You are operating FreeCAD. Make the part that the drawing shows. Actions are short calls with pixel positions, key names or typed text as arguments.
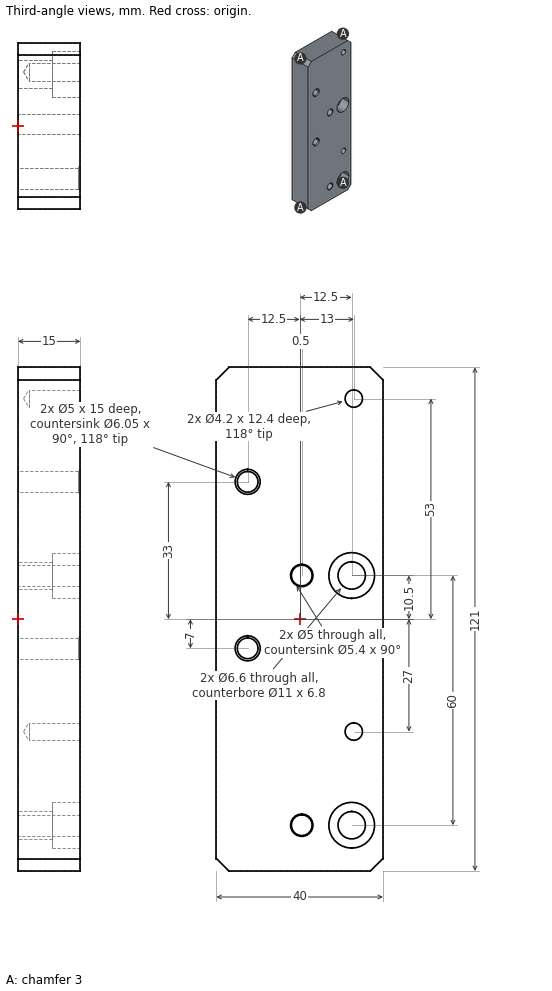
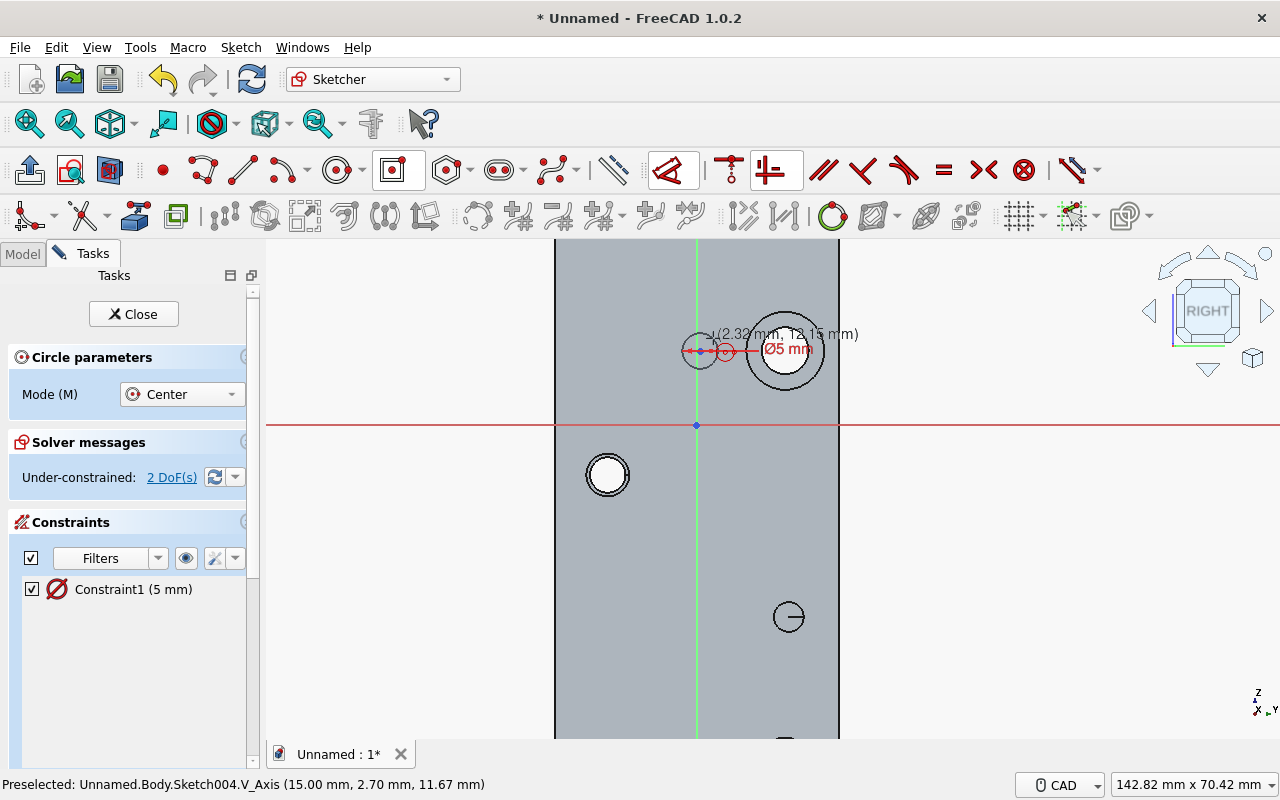
scroll(713, 337, down, 2)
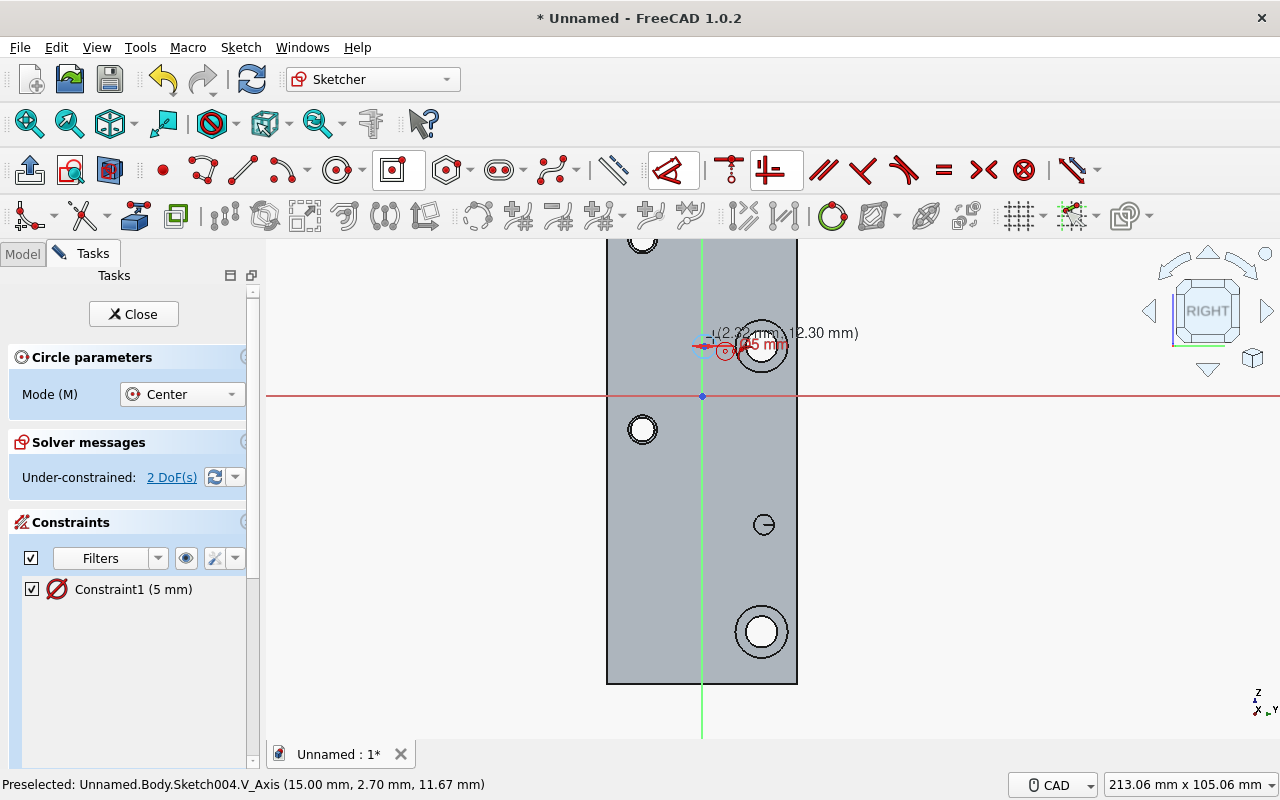
scroll(704, 632, up, 10)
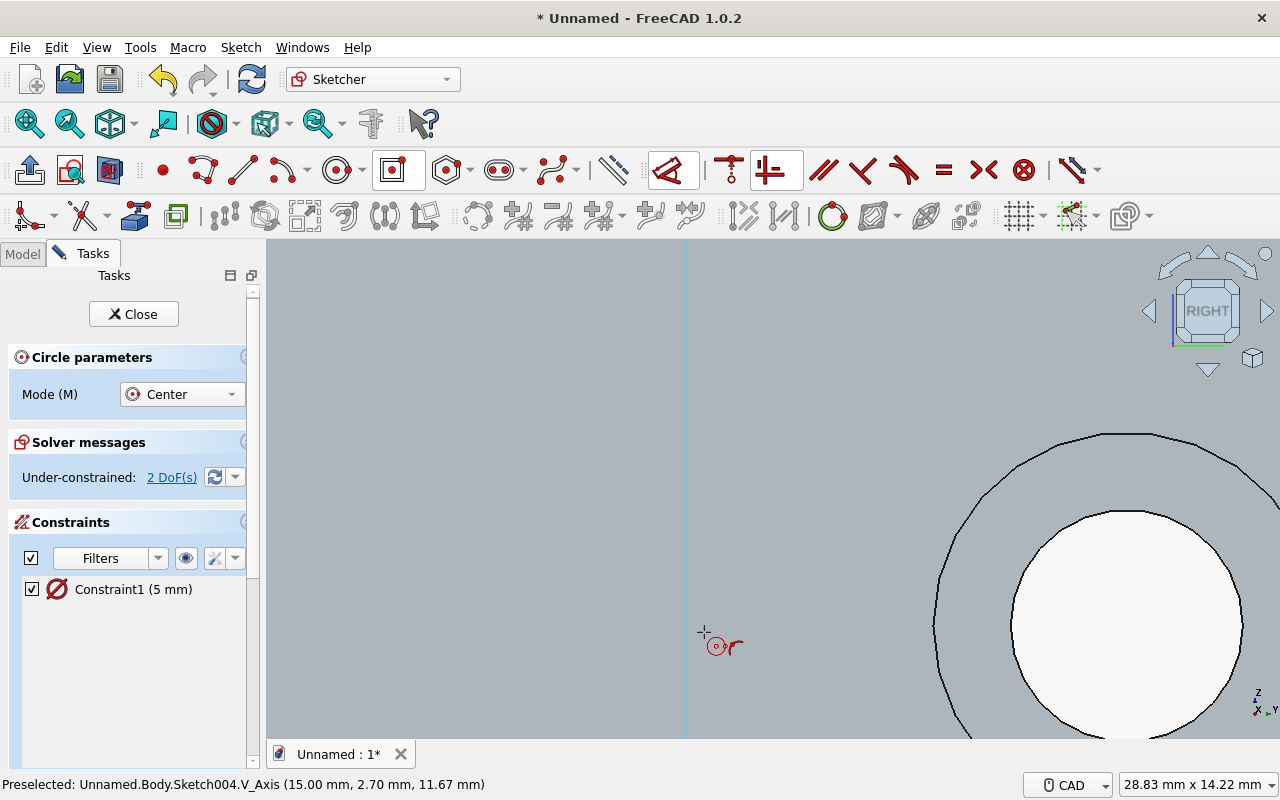
click(705, 626)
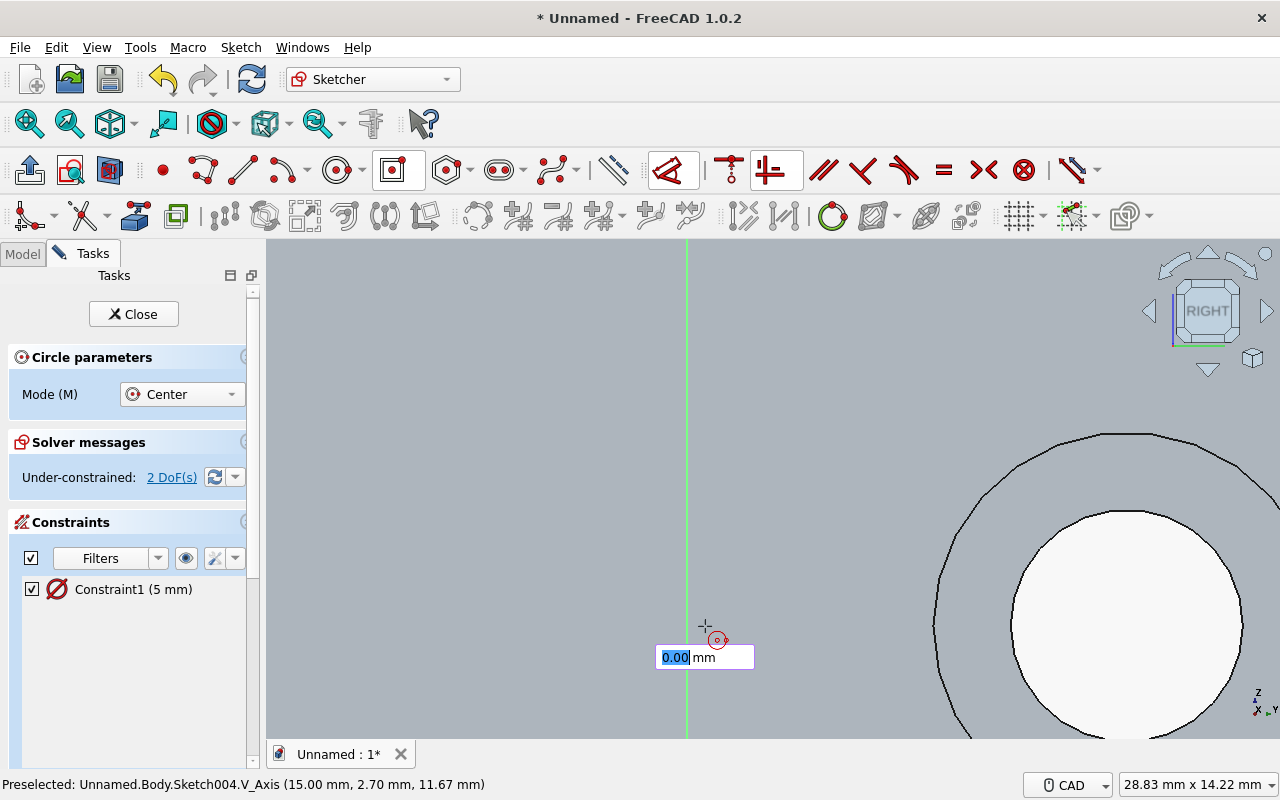
scroll(704, 633, down, 10)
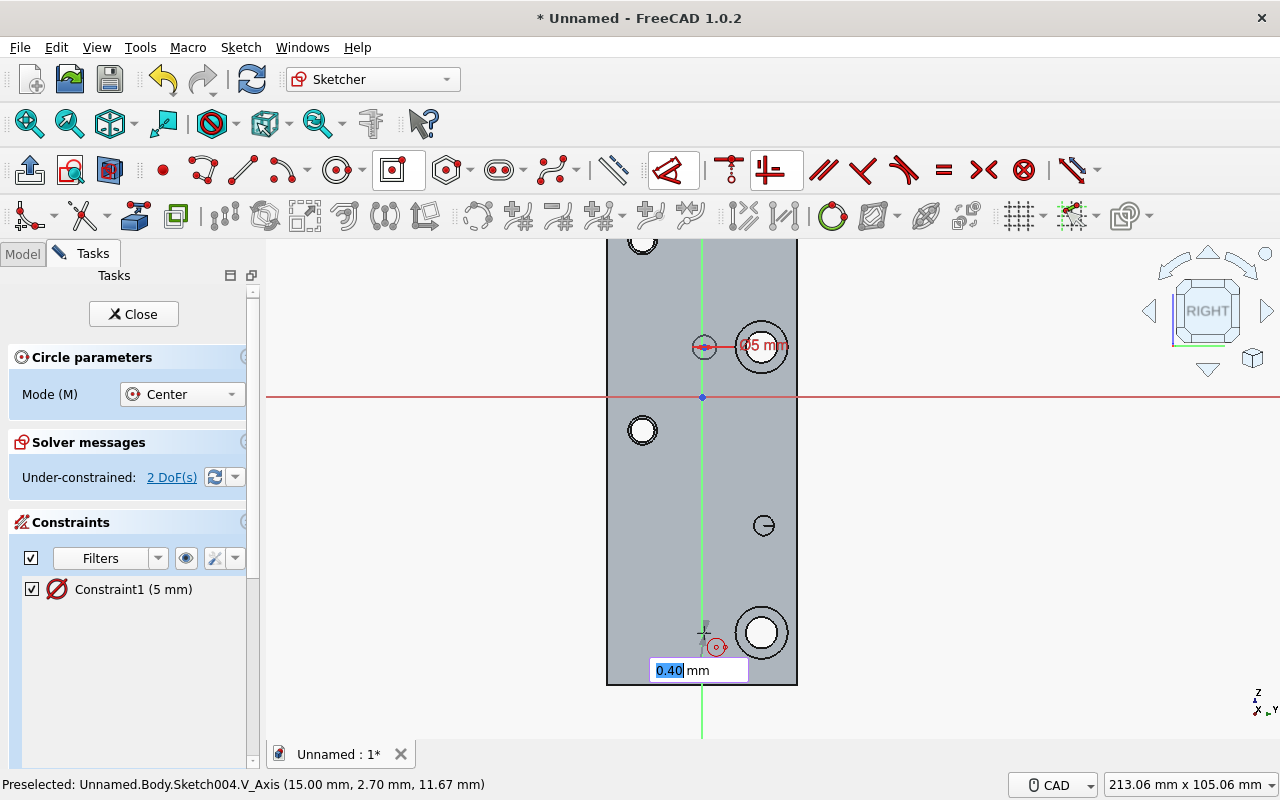
scroll(713, 624, up, 2)
move(713, 624)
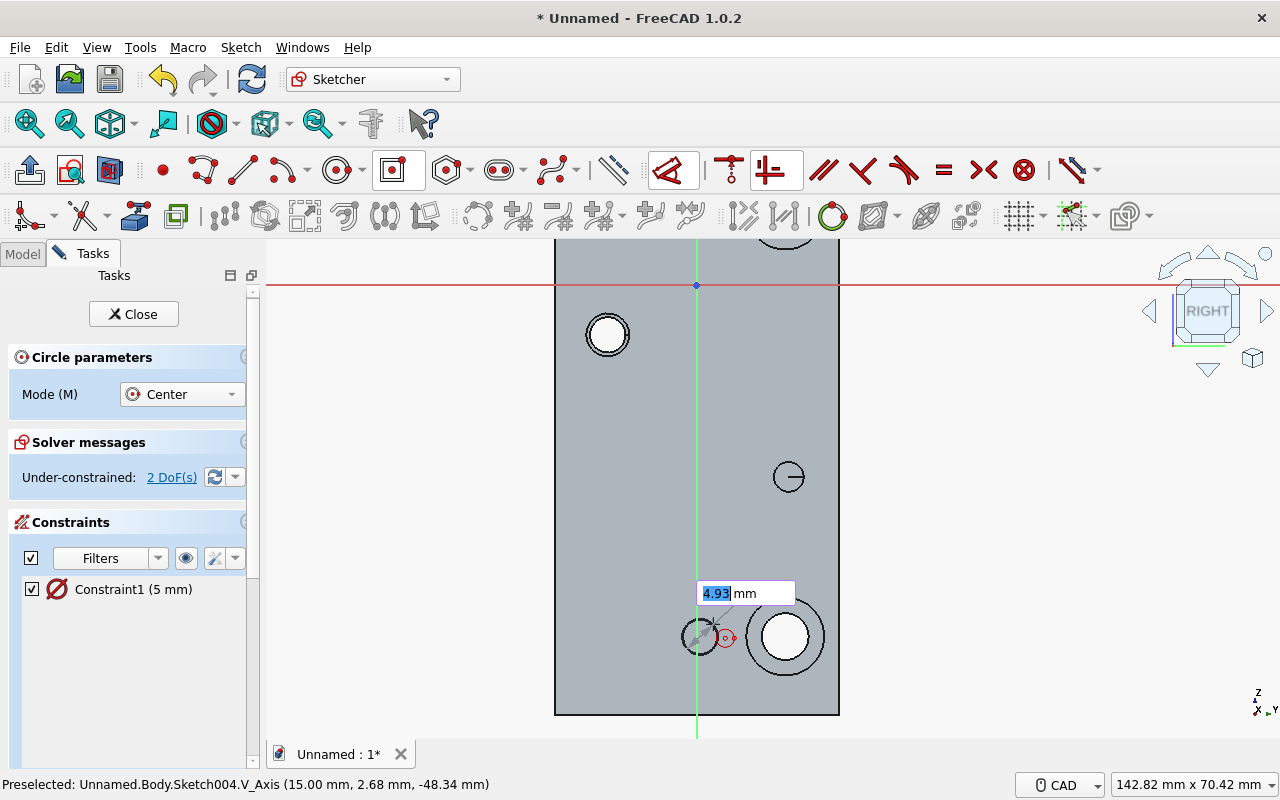
text(5)
key(Return)
key(Escape)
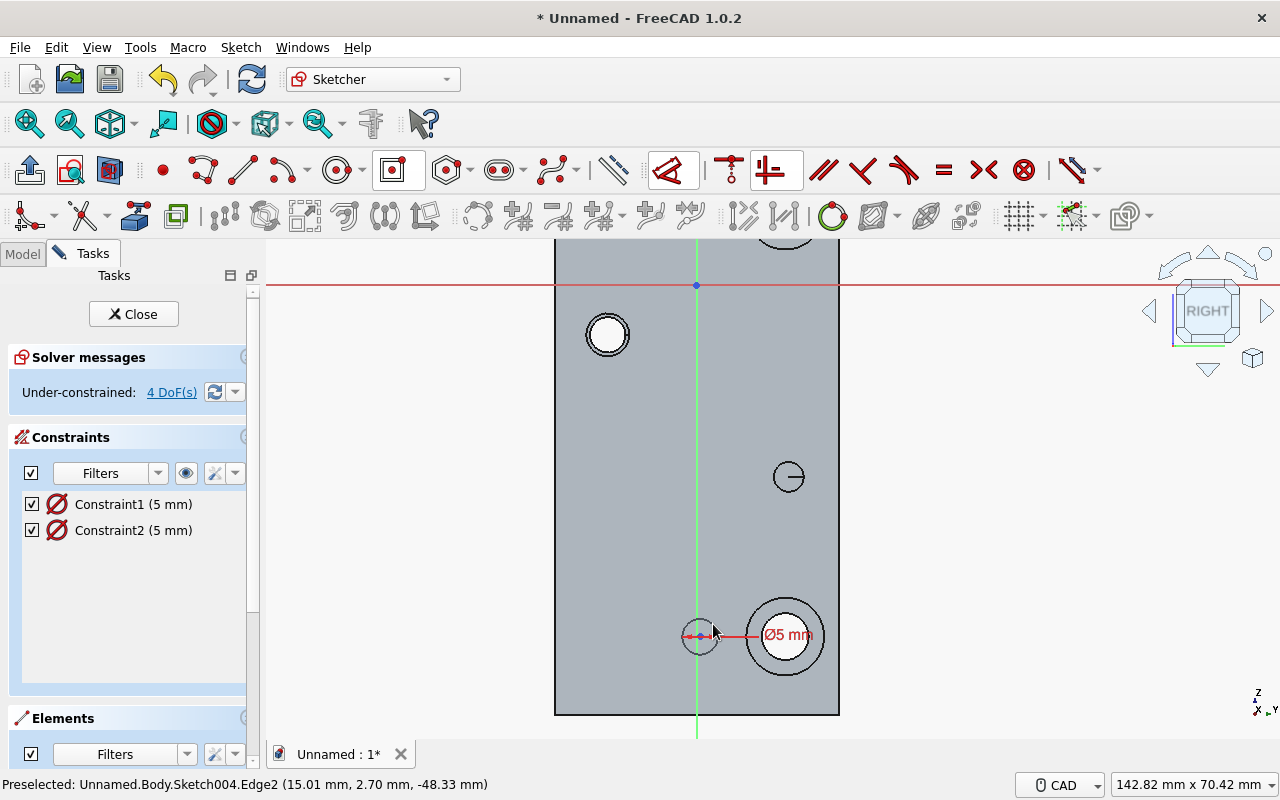
scroll(713, 622, down, 2)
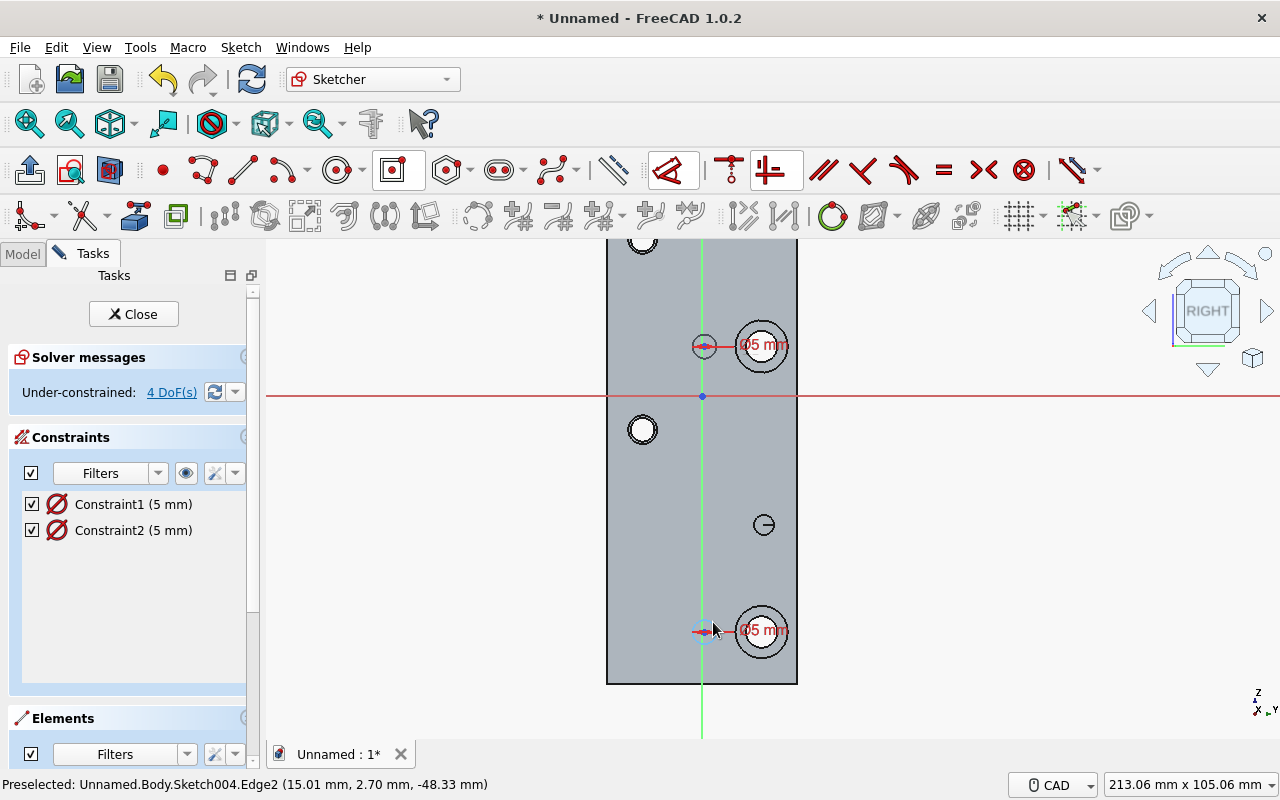
click(705, 347)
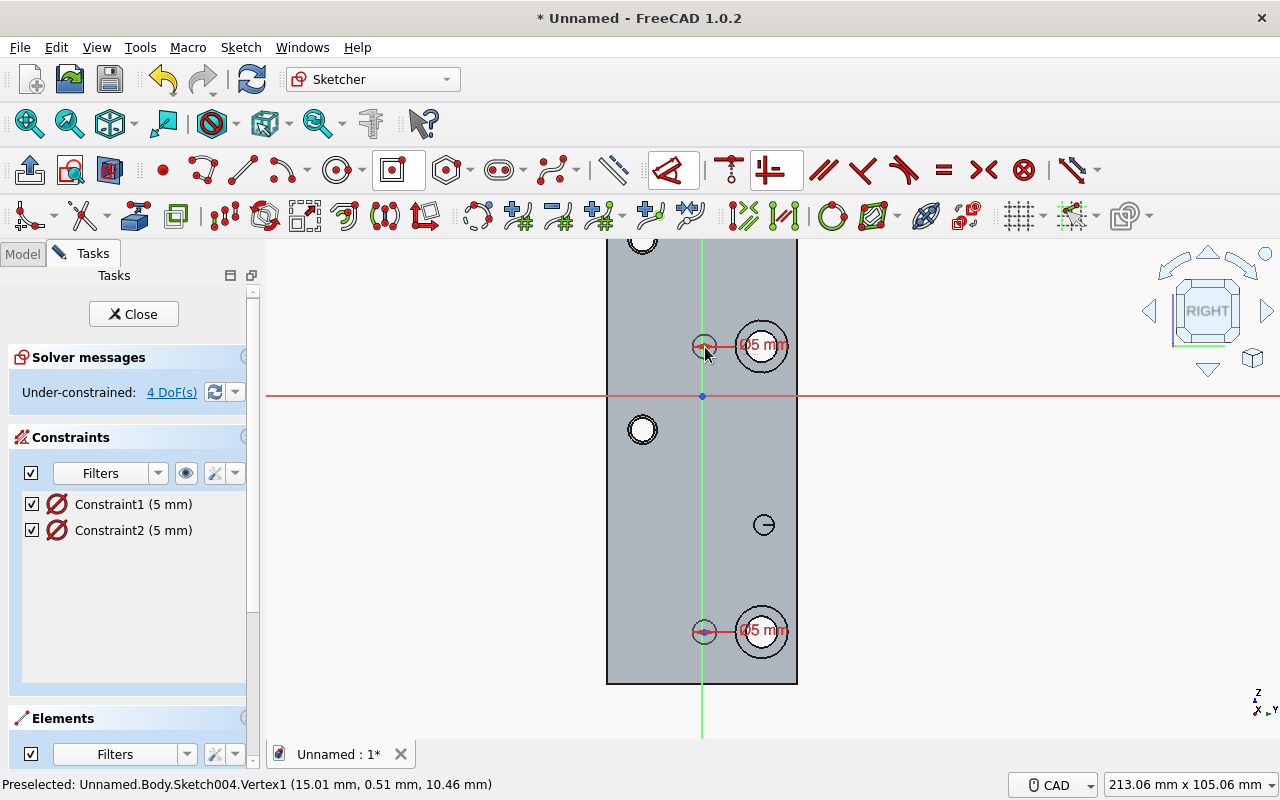
click(705, 632)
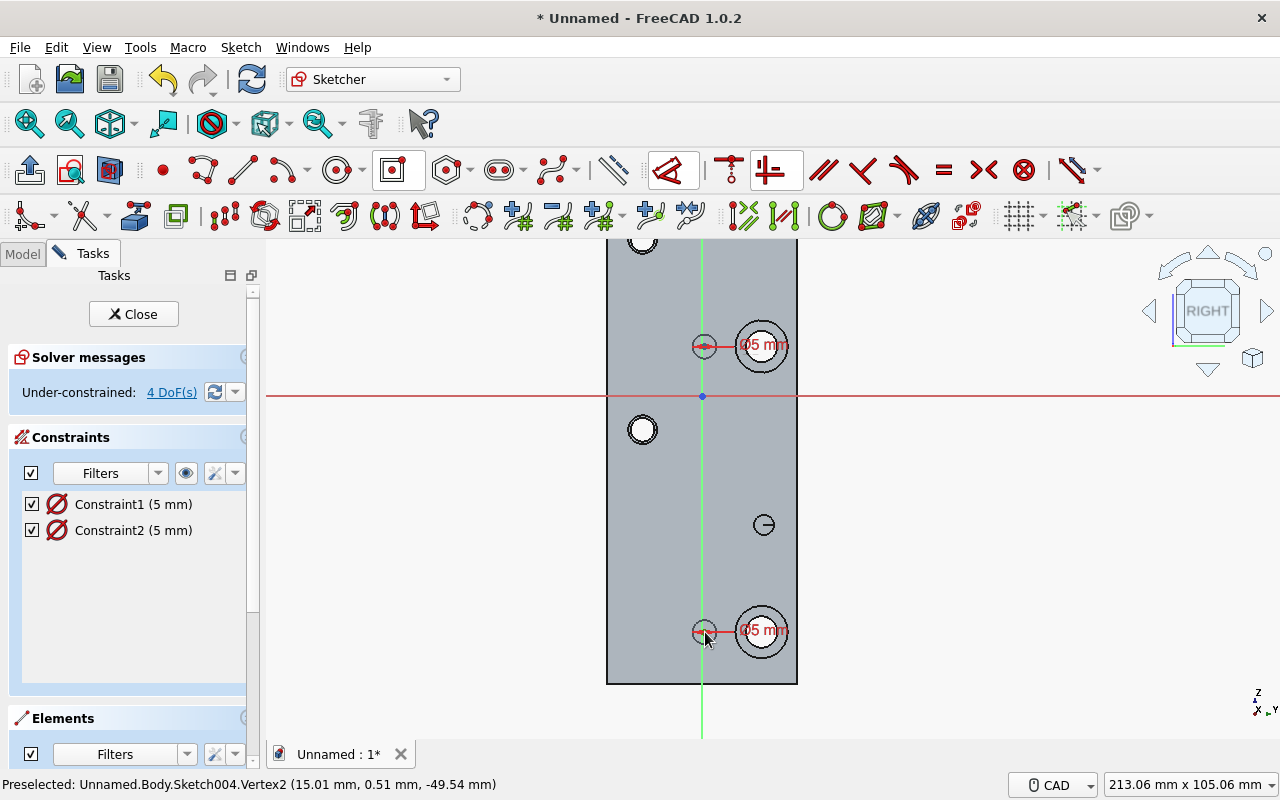
click(798, 170)